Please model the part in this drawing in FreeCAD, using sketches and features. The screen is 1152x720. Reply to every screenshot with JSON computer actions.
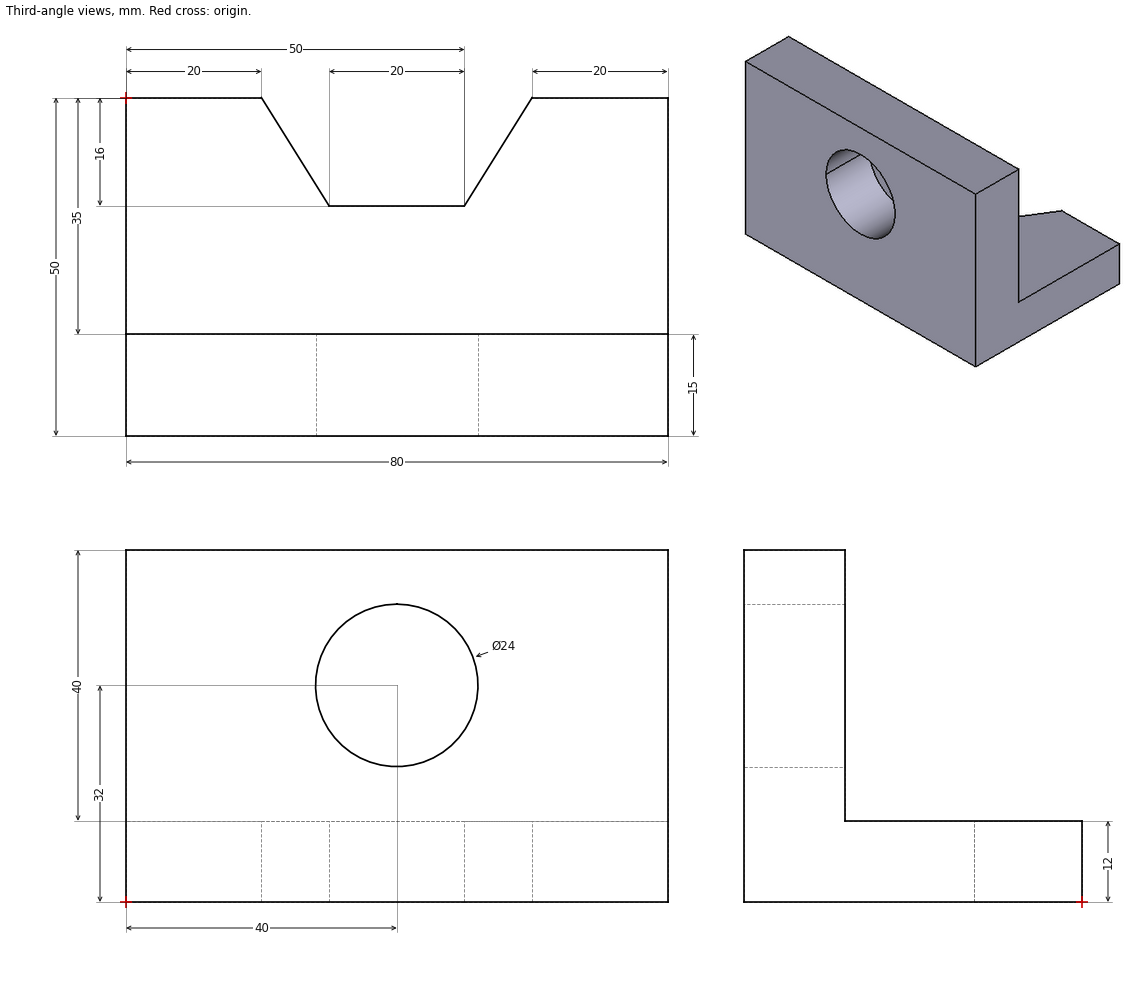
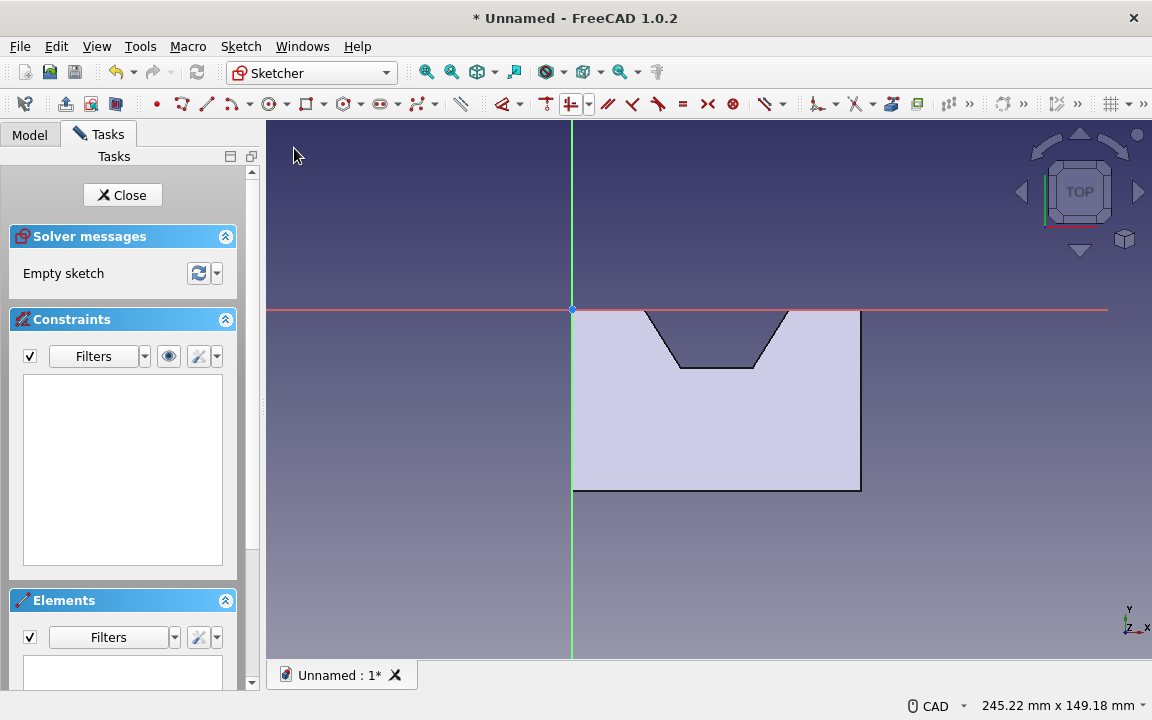
{"action": "scroll", "coordinate": [809, 413], "scroll_direction": "up", "scroll_amount": 3}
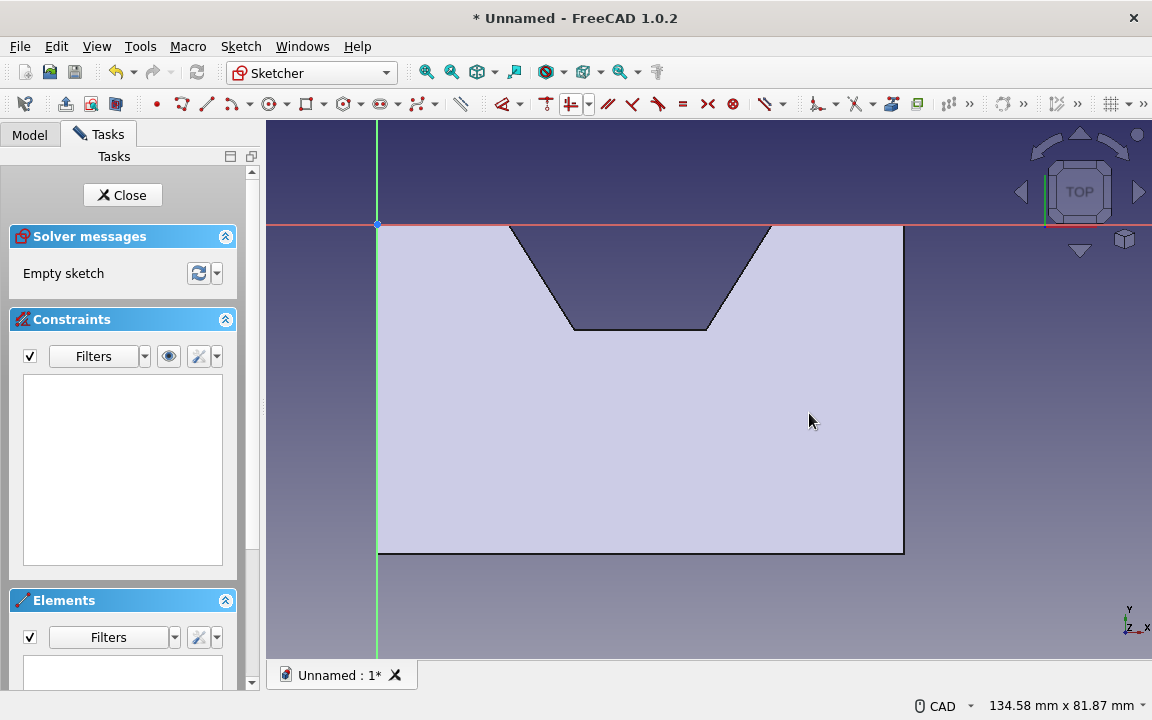
{"action": "left_click", "coordinate": [306, 104]}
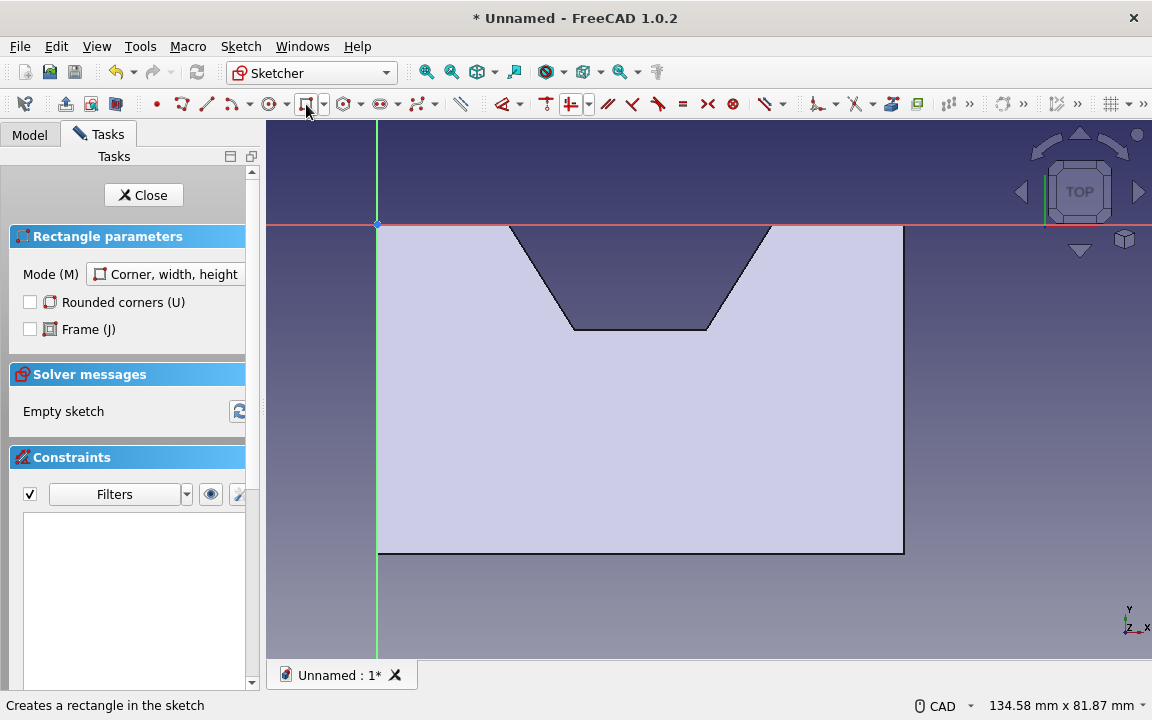
{"action": "left_click", "coordinate": [377, 455]}
{"action": "mouse_move", "coordinate": [904, 554]}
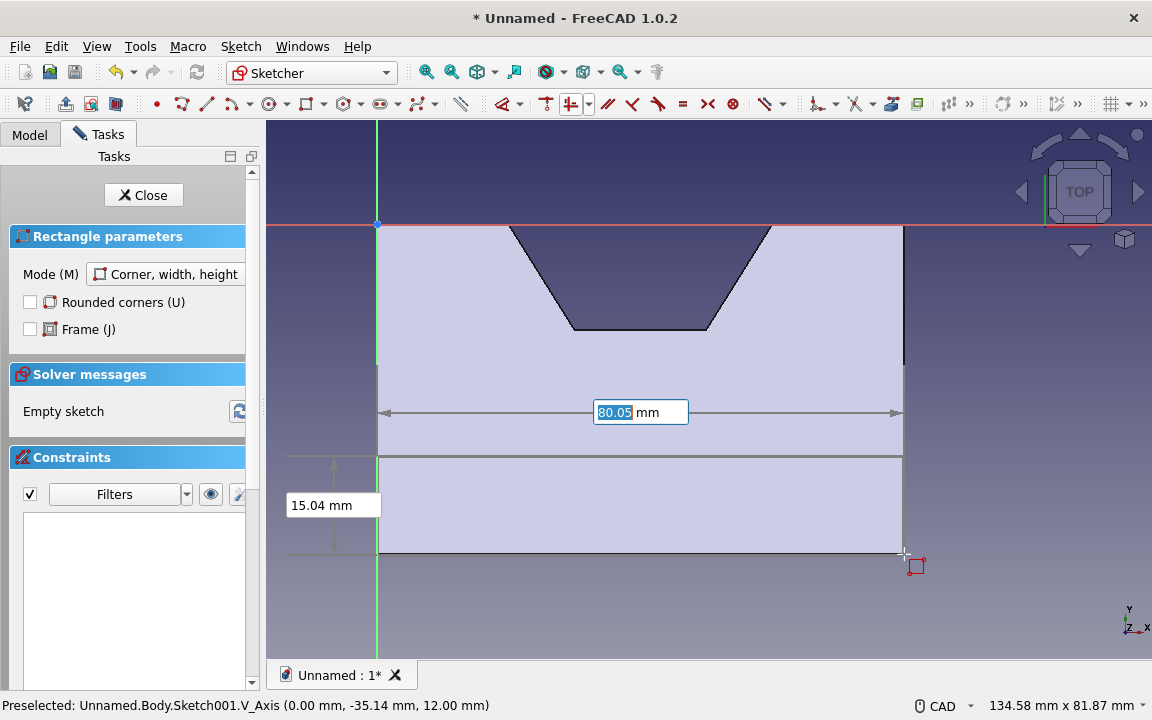
{"action": "type", "text": "80"}
{"action": "key", "text": "Tab"}
{"action": "type", "text": "15"}
{"action": "key", "text": "Return"}
{"action": "key", "text": "Escape"}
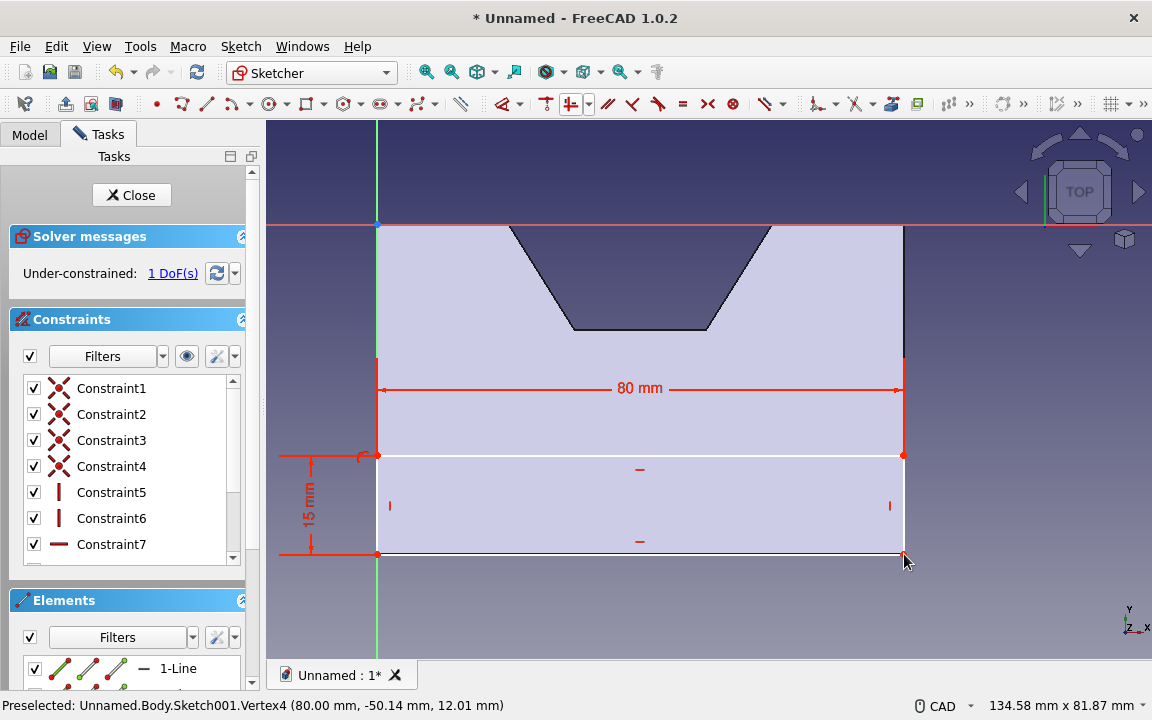
{"action": "left_click", "coordinate": [502, 104]}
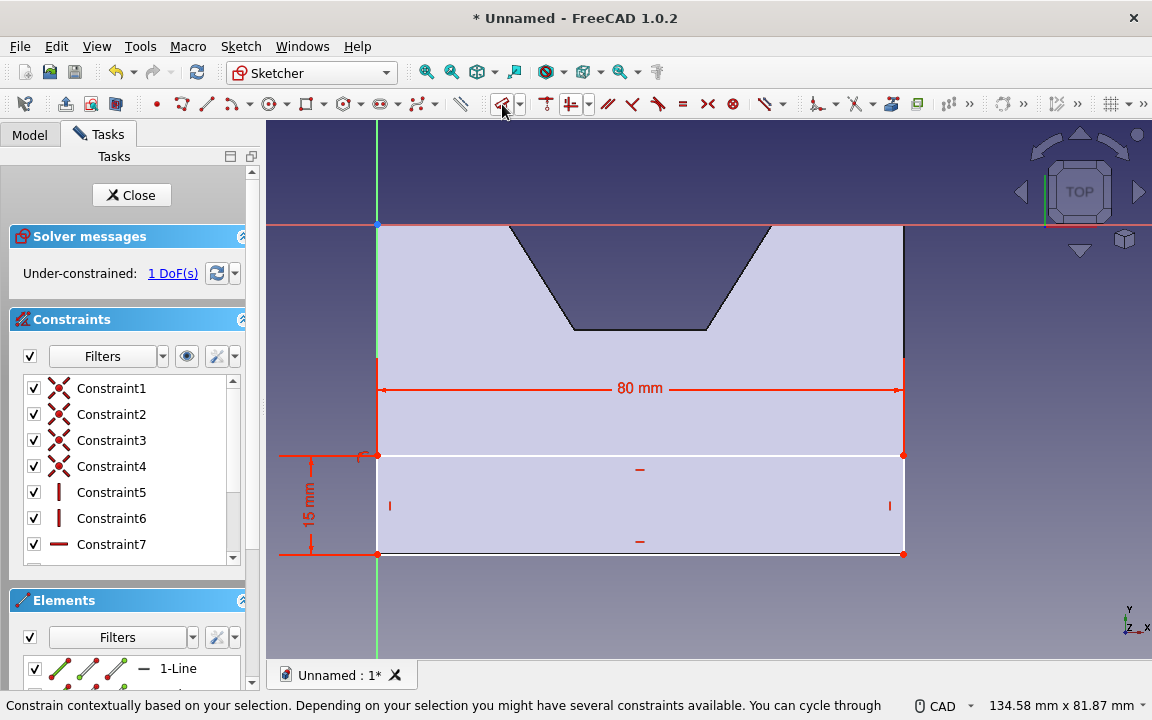
{"action": "left_click", "coordinate": [377, 456]}
{"action": "left_click", "coordinate": [343, 340]}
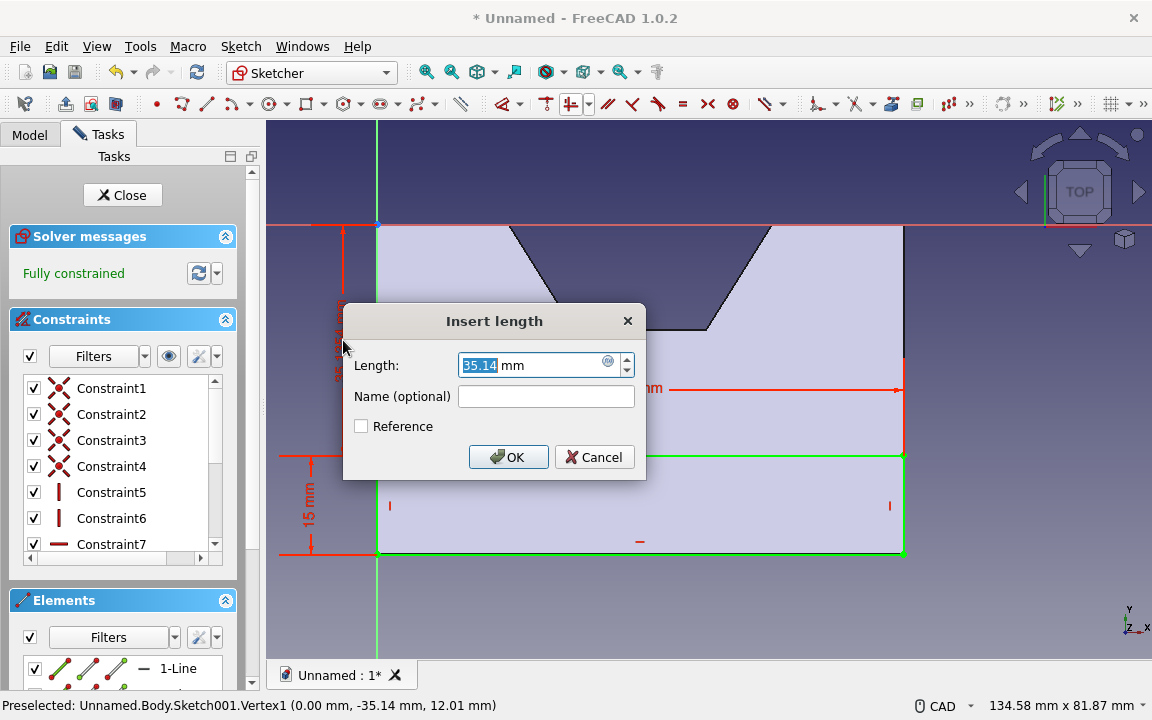
{"action": "type", "text": "35"}
{"action": "key", "text": "Return"}
{"action": "key", "text": "Escape"}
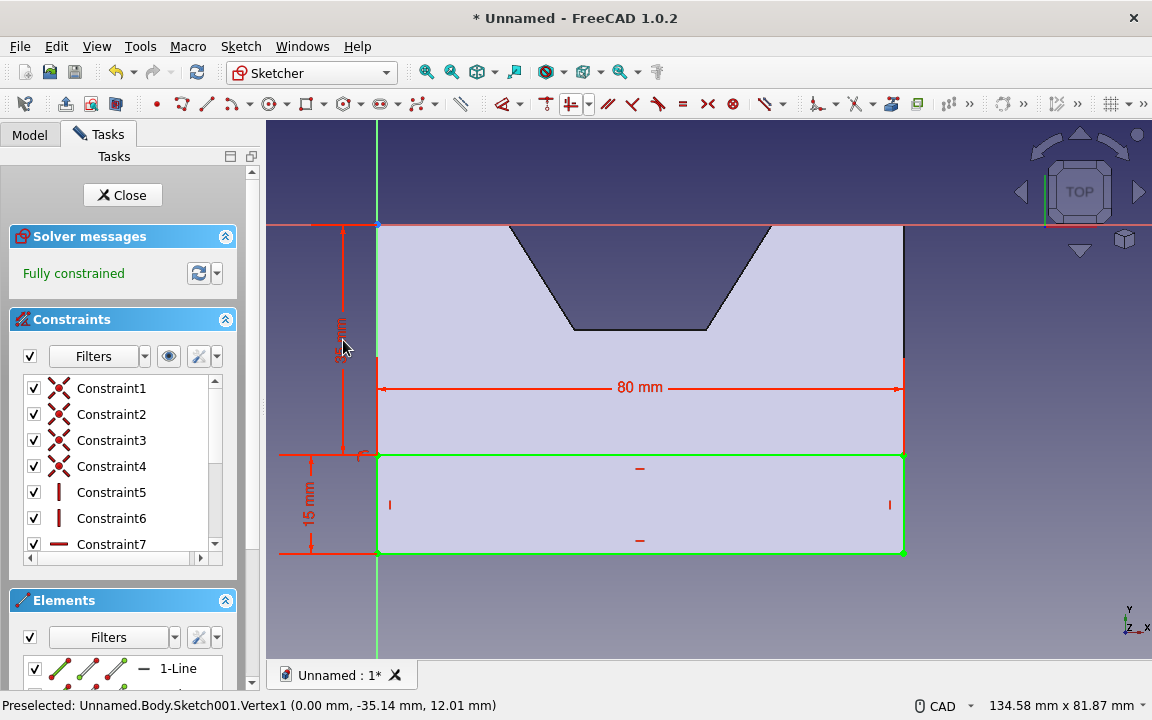
{"action": "left_click", "coordinate": [123, 195]}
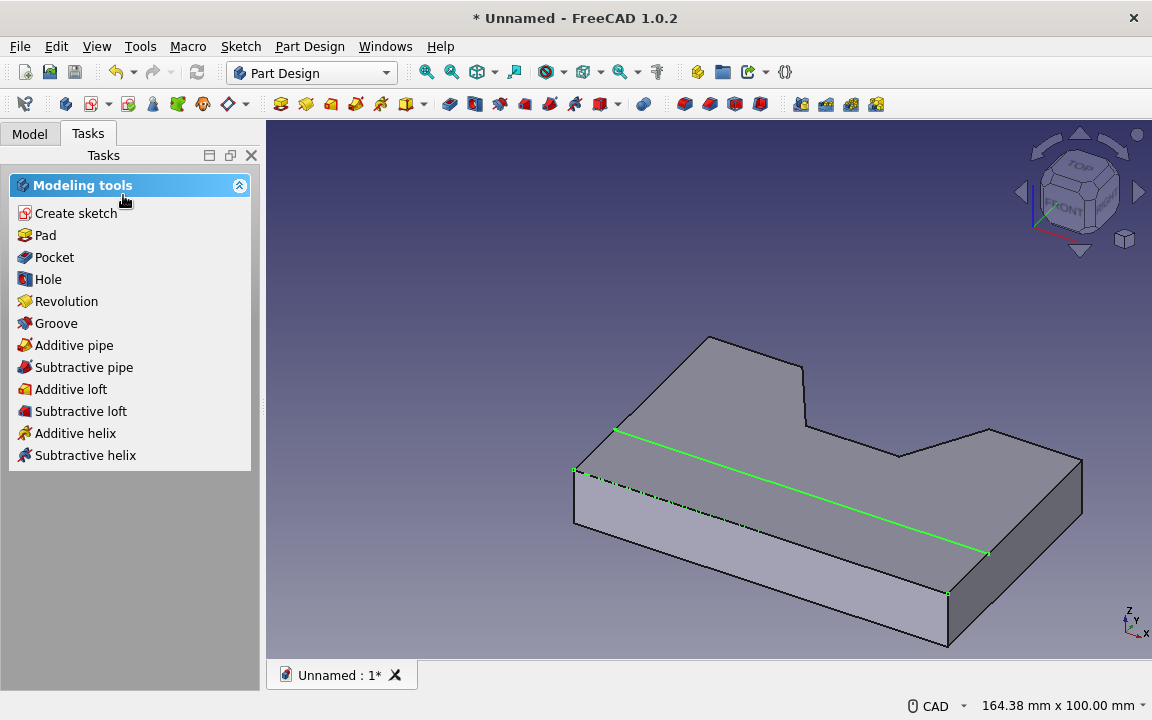
{"action": "left_click", "coordinate": [281, 104]}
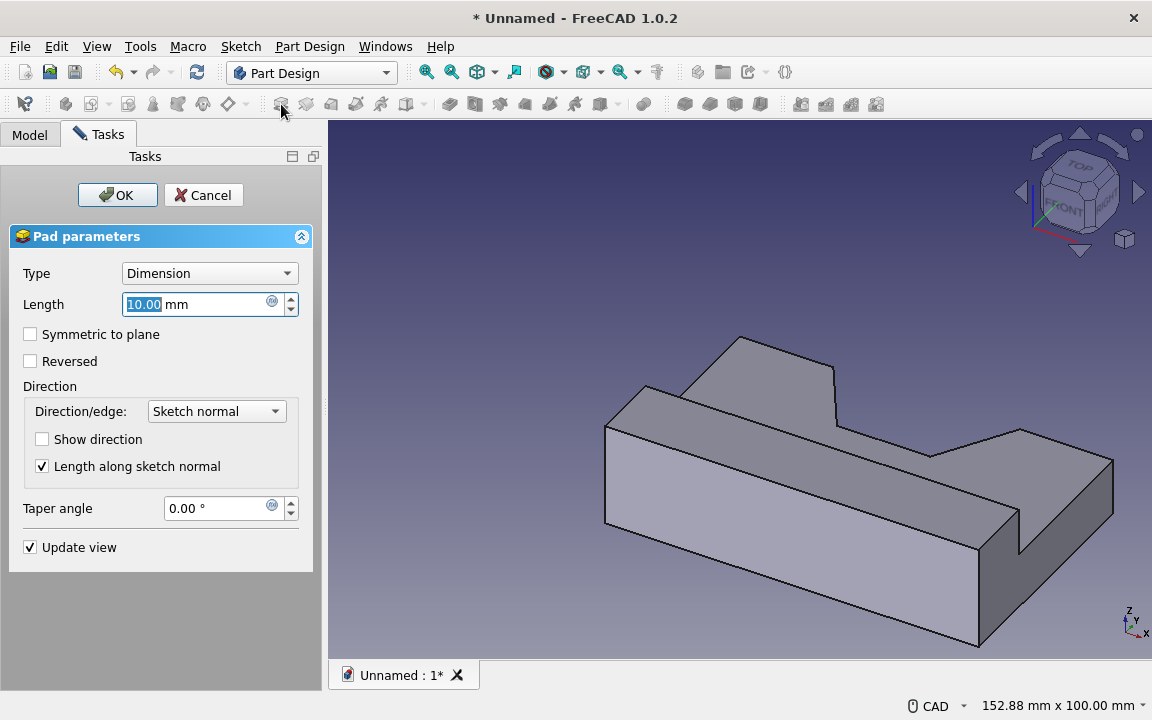
{"action": "type", "text": "40"}
{"action": "key", "text": "Tab"}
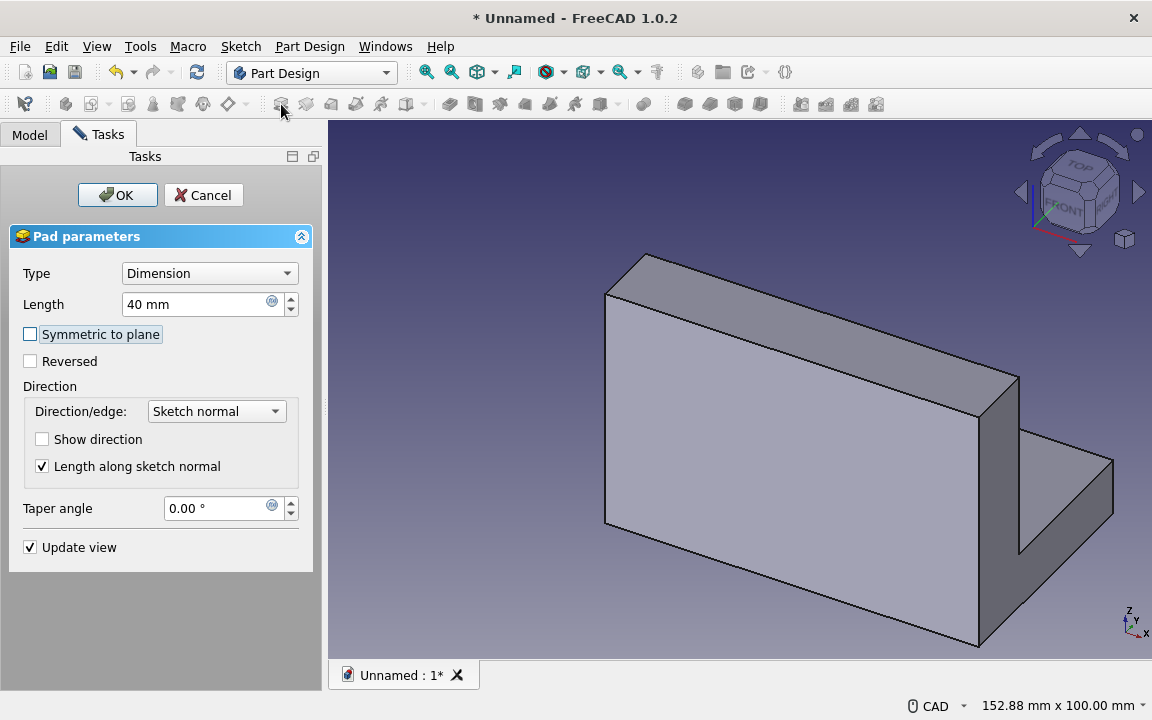
{"action": "left_click", "coordinate": [118, 195]}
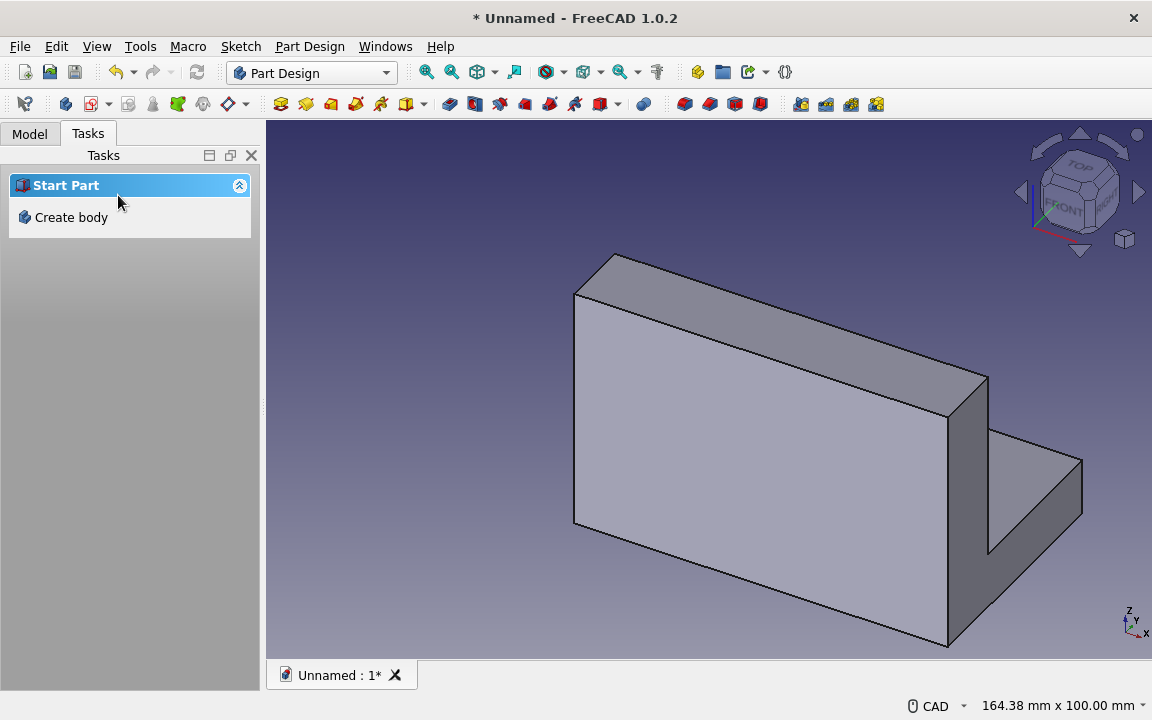
{"action": "key", "text": "4"}